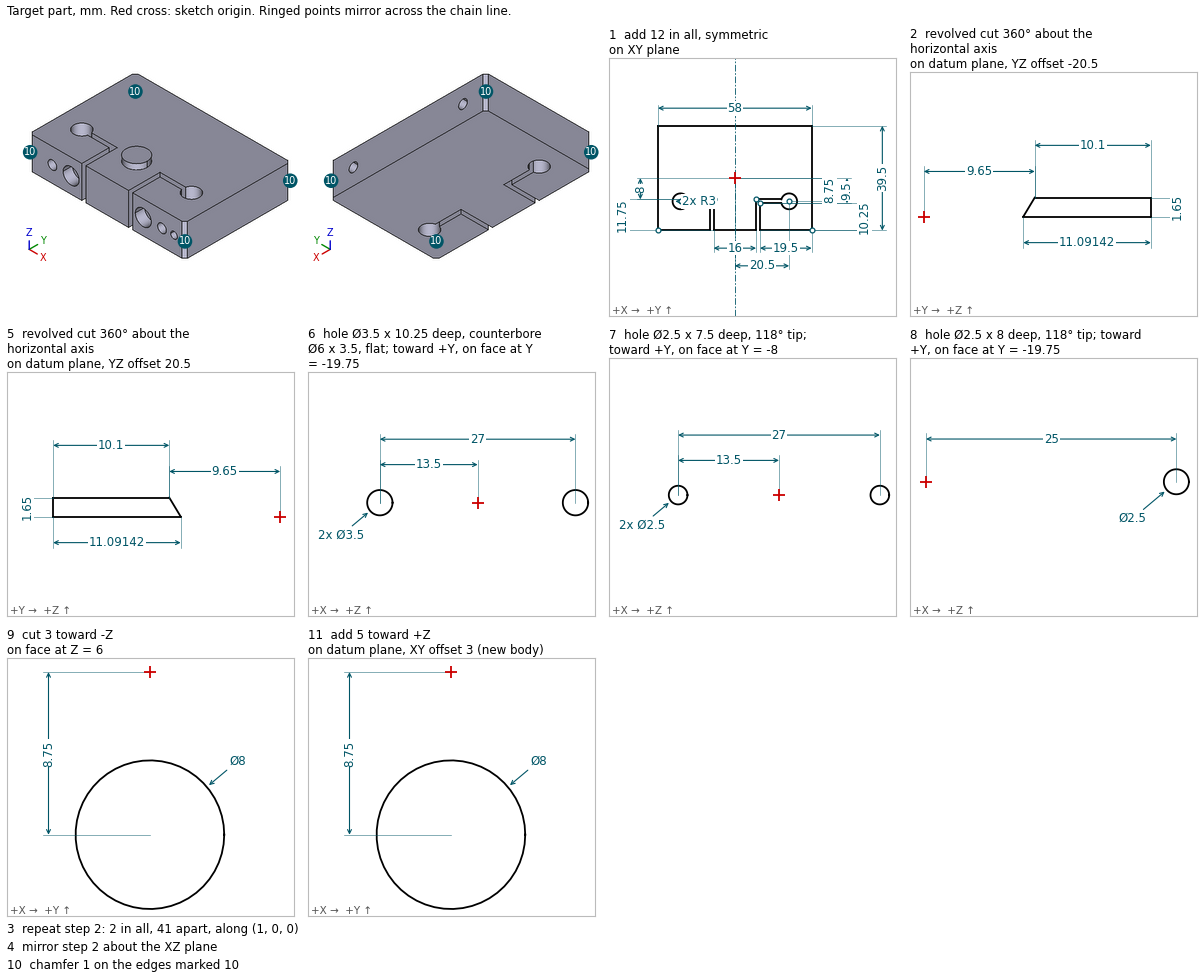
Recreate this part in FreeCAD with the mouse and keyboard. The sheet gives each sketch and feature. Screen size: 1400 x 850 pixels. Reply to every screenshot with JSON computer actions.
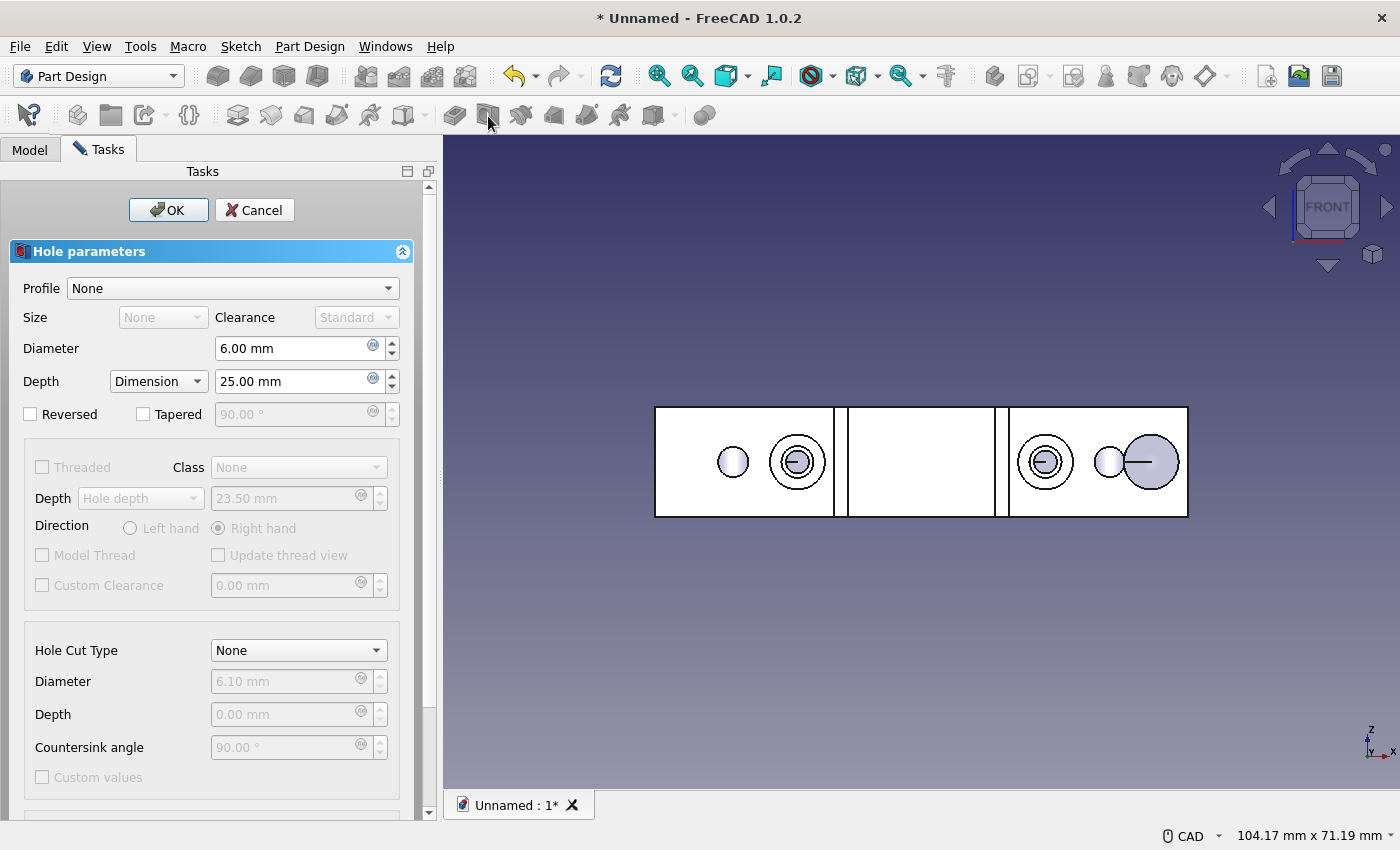
{"action": "triple_click", "coordinate": [300, 348]}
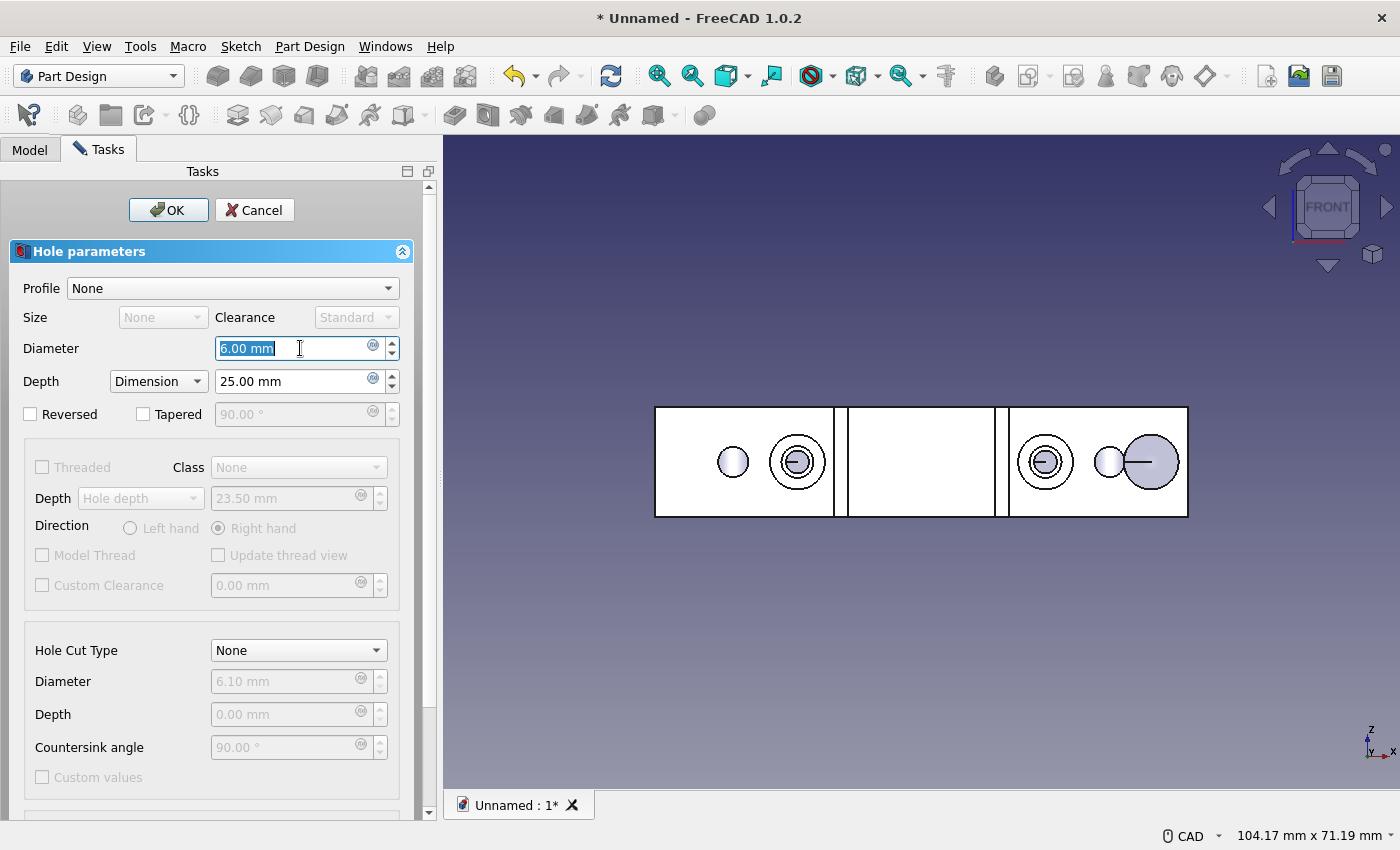
{"action": "type", "text": "2.5"}
{"action": "key", "text": "Tab"}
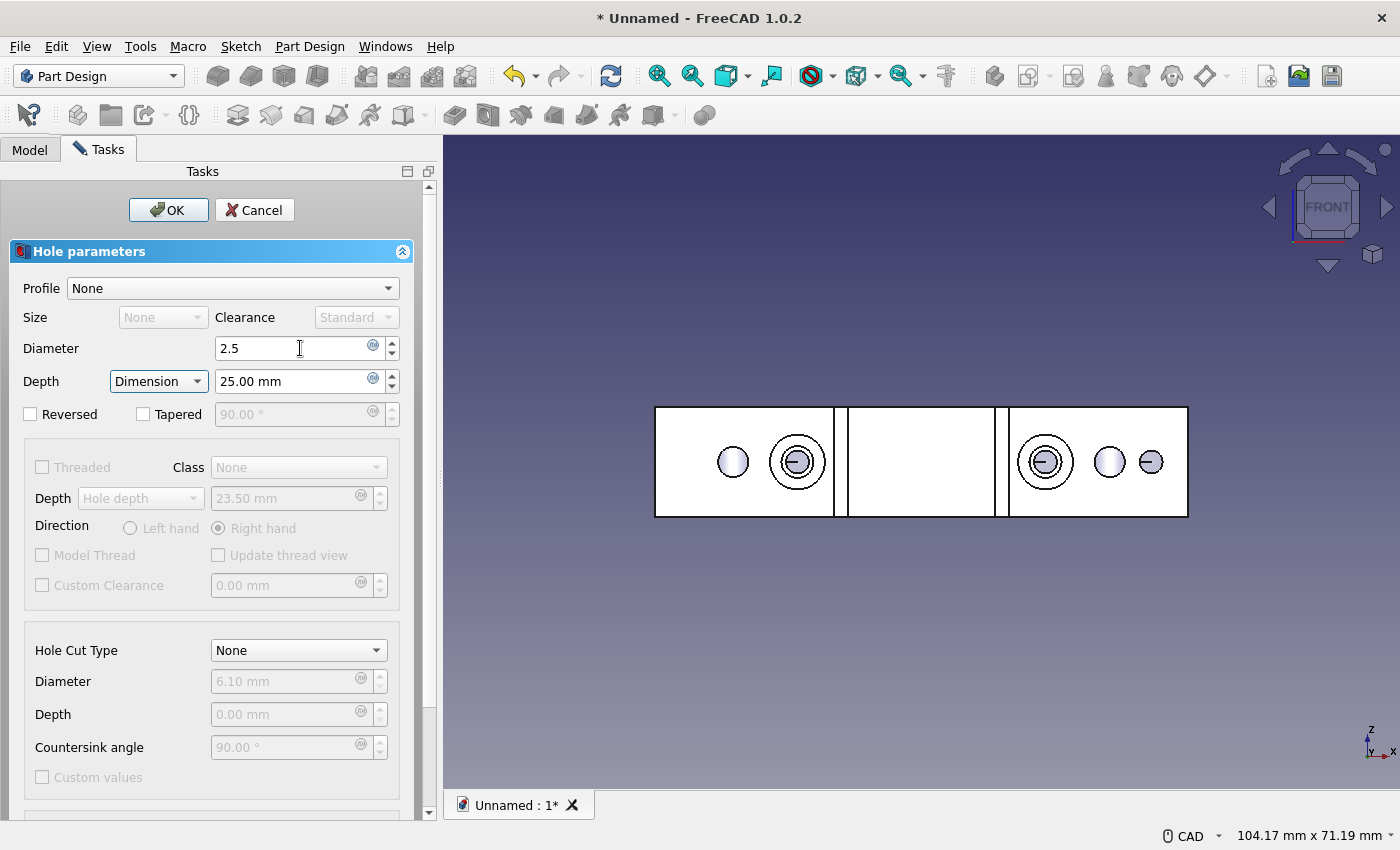
{"action": "triple_click", "coordinate": [300, 382]}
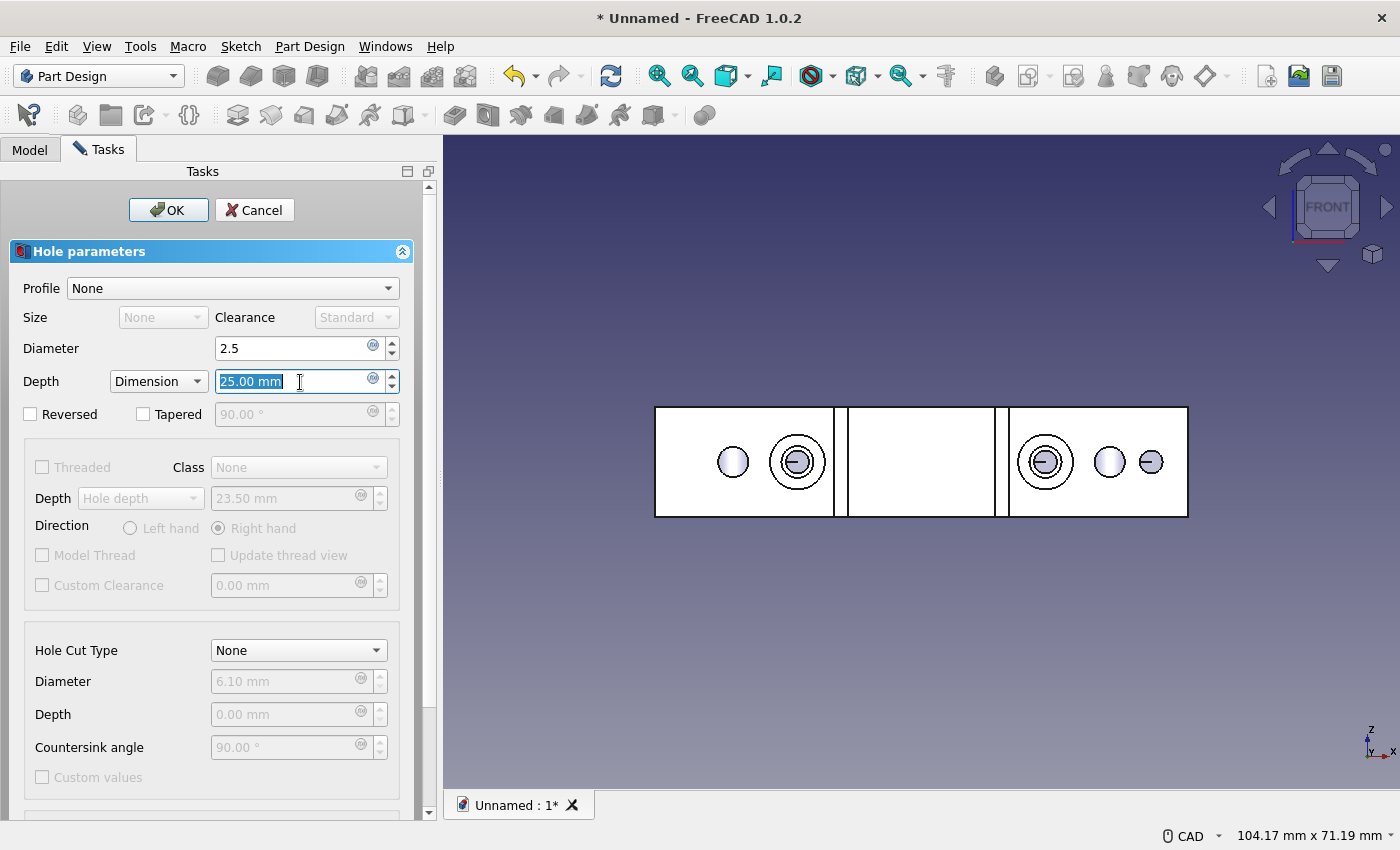
{"action": "type", "text": "8"}
{"action": "key", "text": "Tab"}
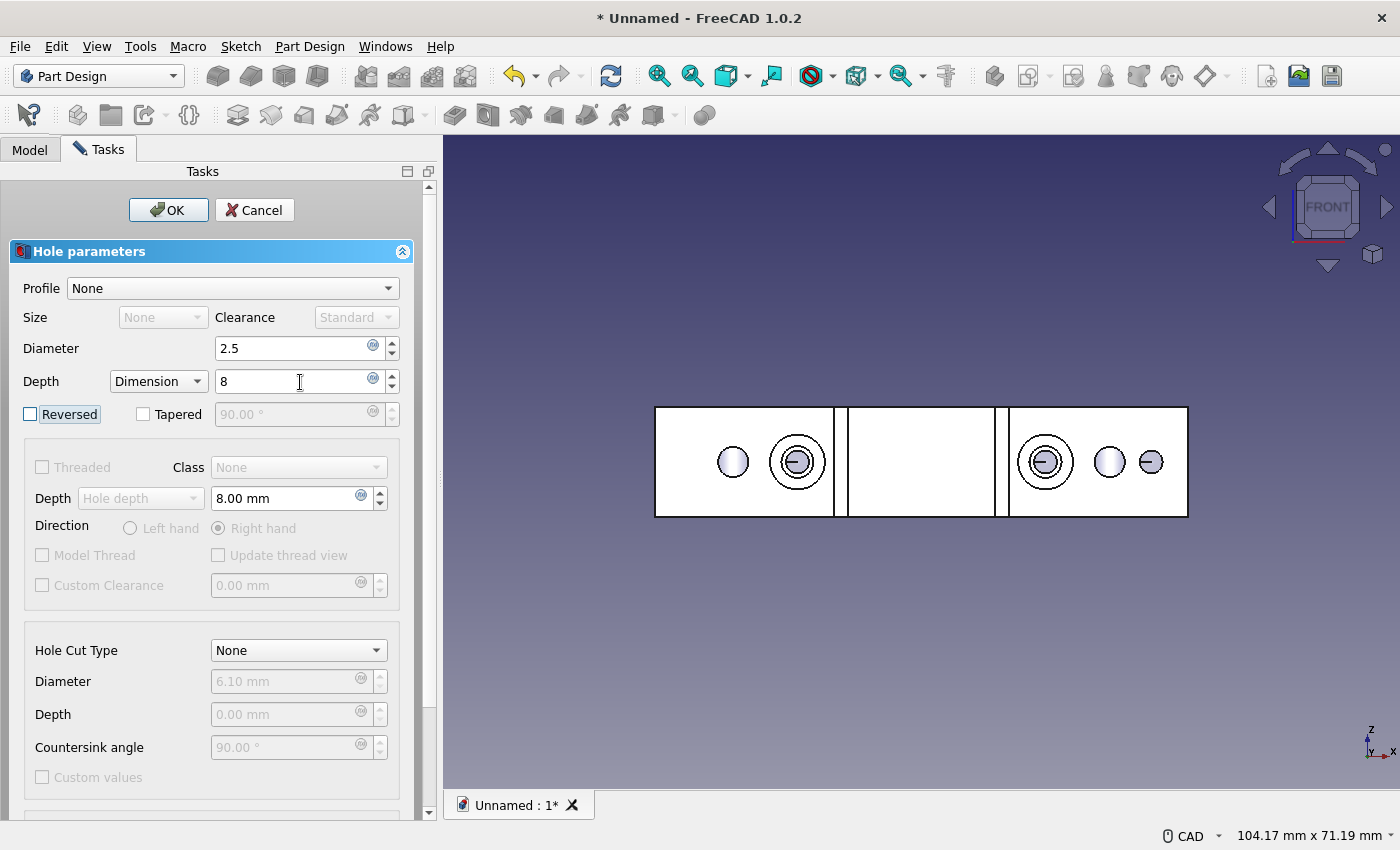
{"action": "left_click", "coordinate": [169, 210]}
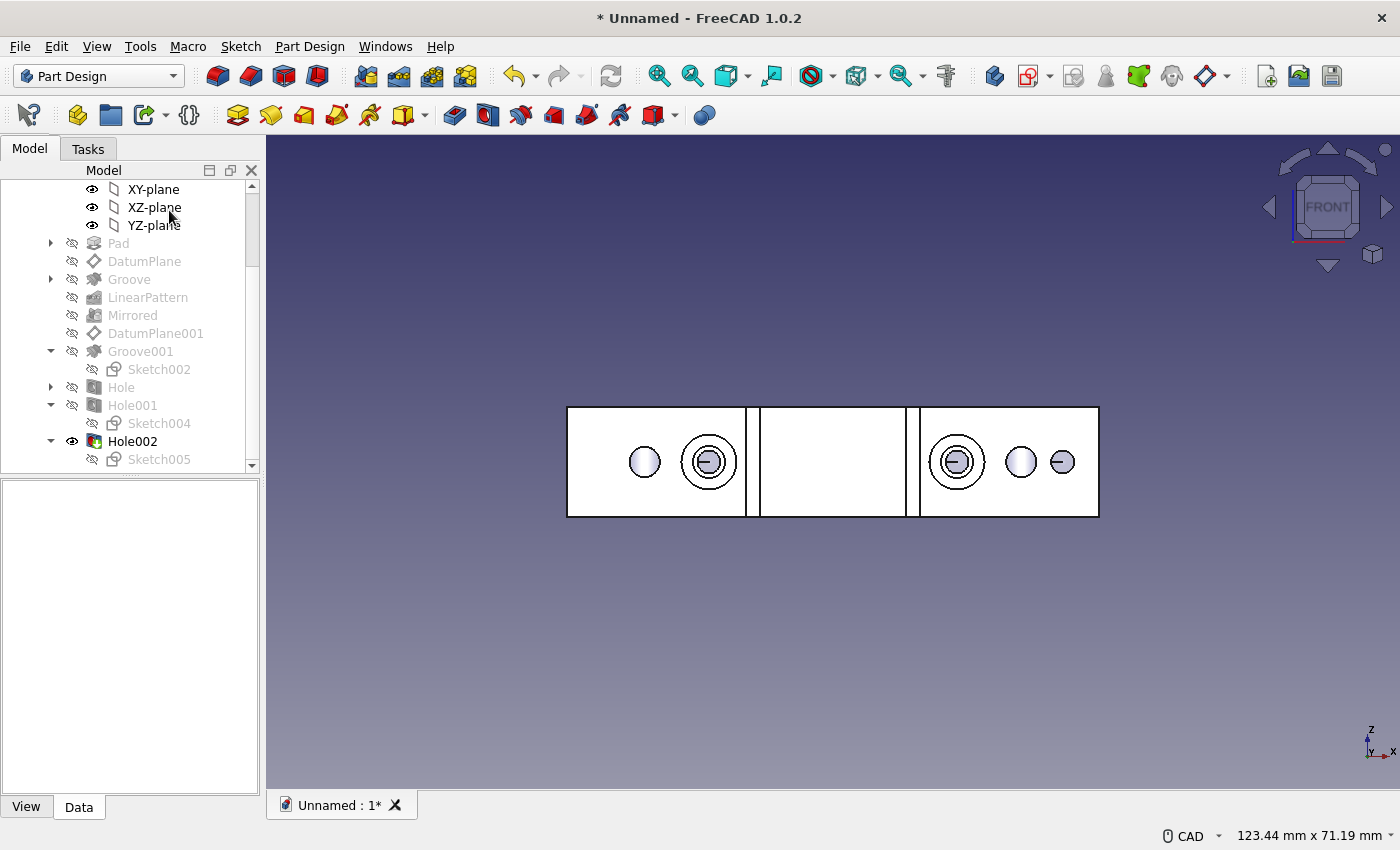
{"action": "key", "text": "0"}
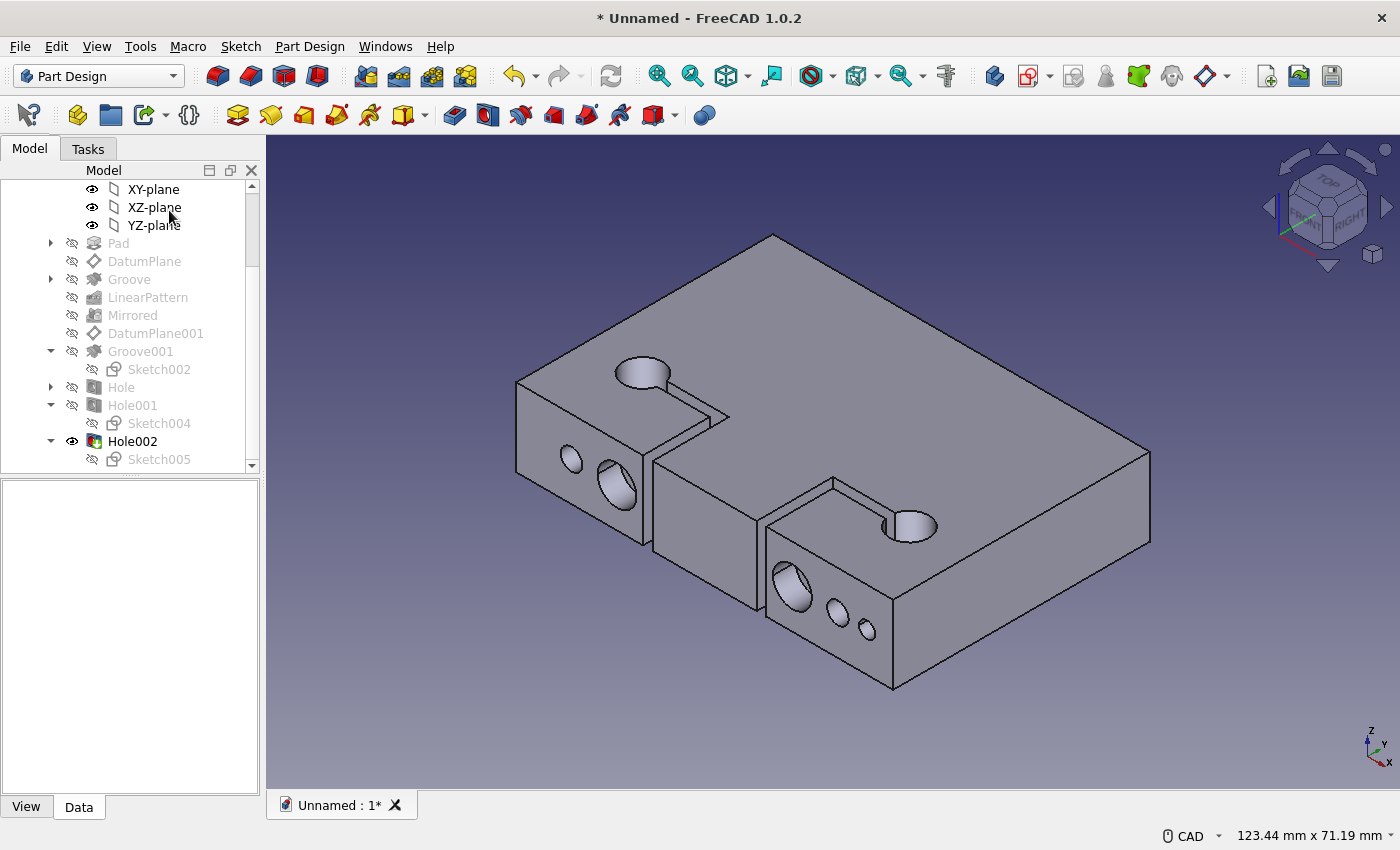
{"action": "left_click", "coordinate": [870, 395]}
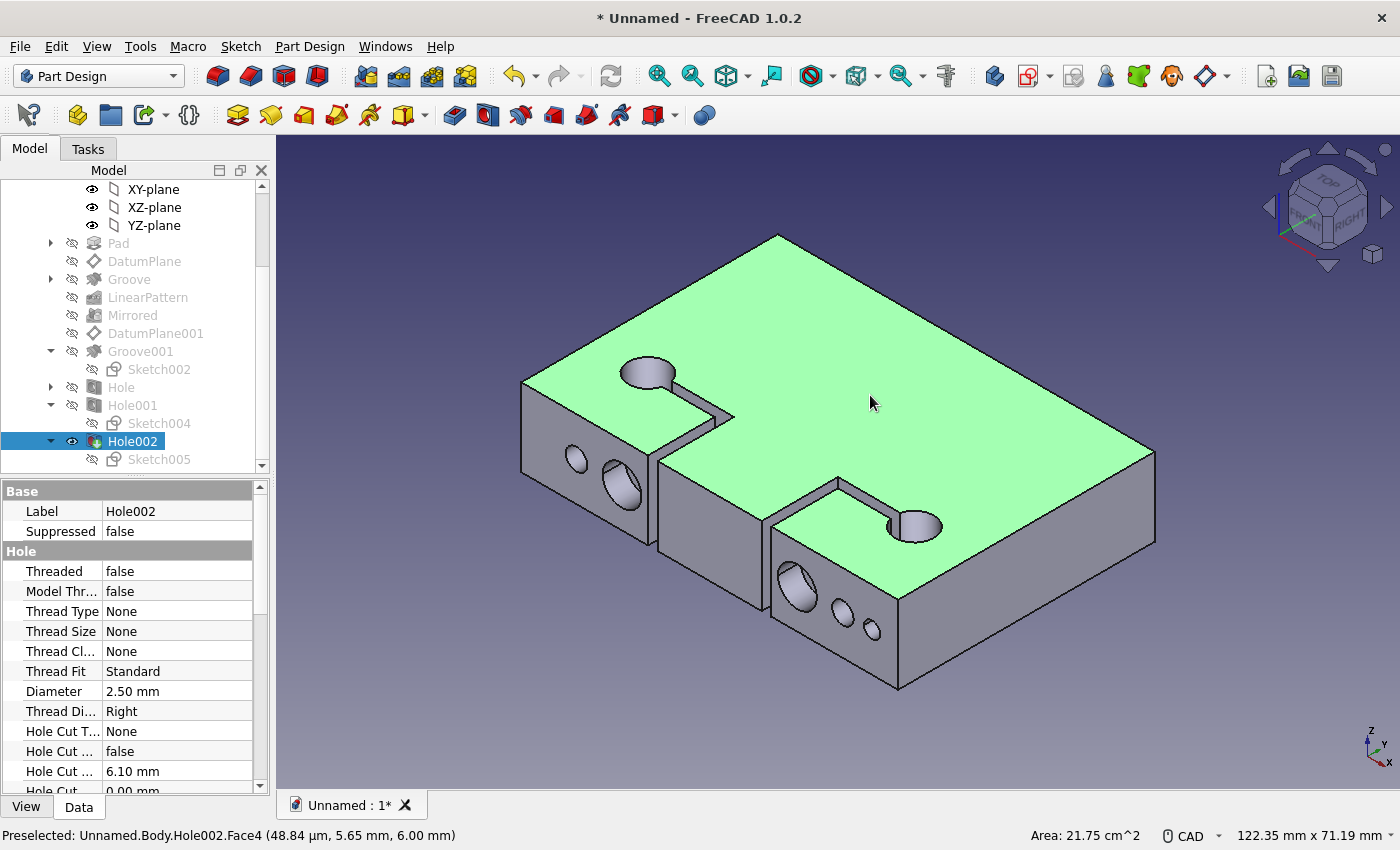
{"action": "left_click", "coordinate": [1028, 76]}